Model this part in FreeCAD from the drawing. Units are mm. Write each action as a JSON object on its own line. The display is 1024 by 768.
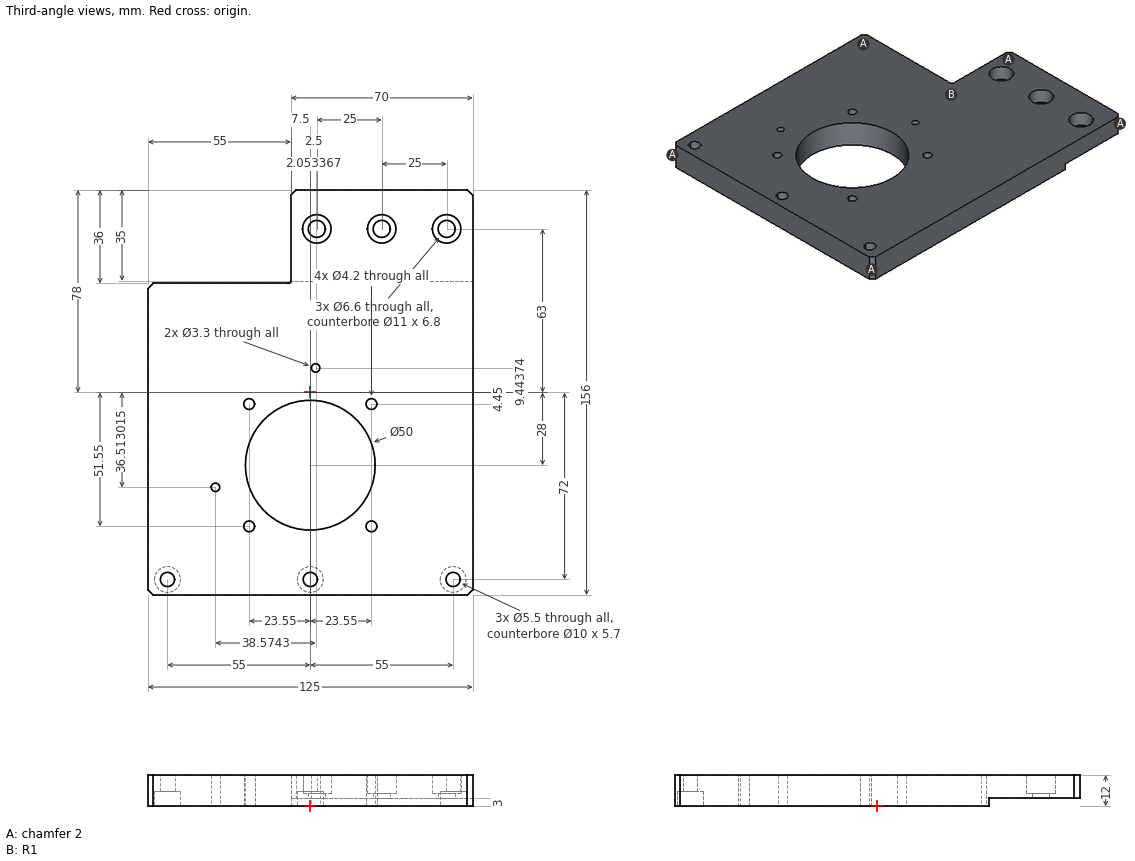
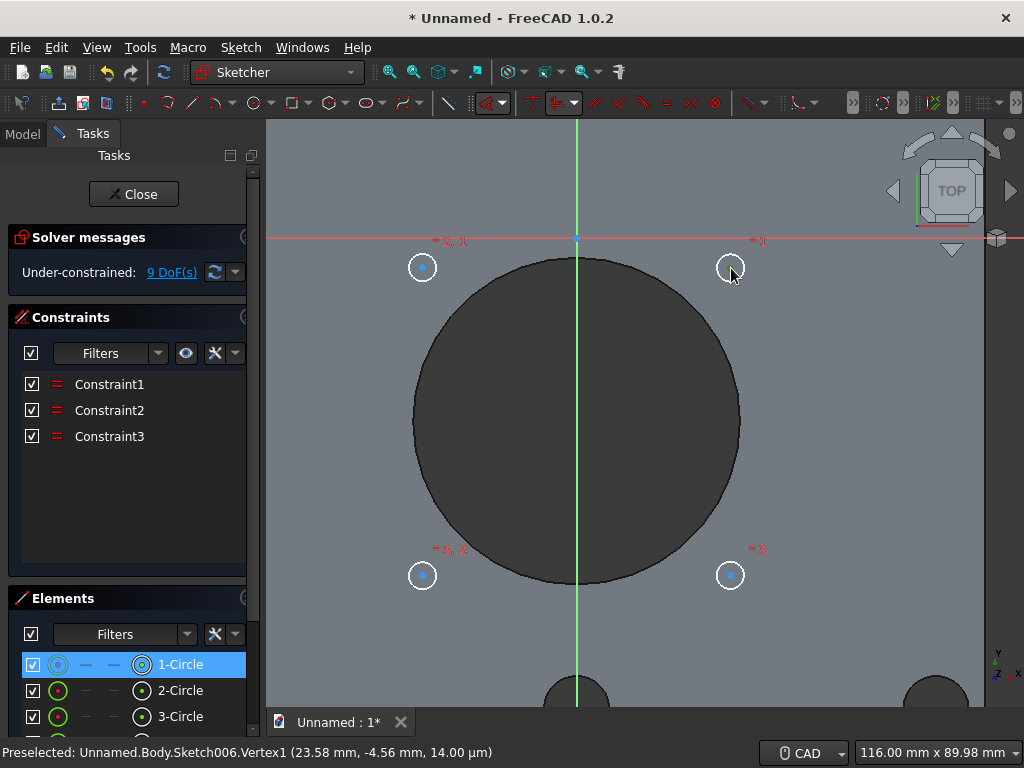
{"action": "left_click", "coordinate": [423, 268]}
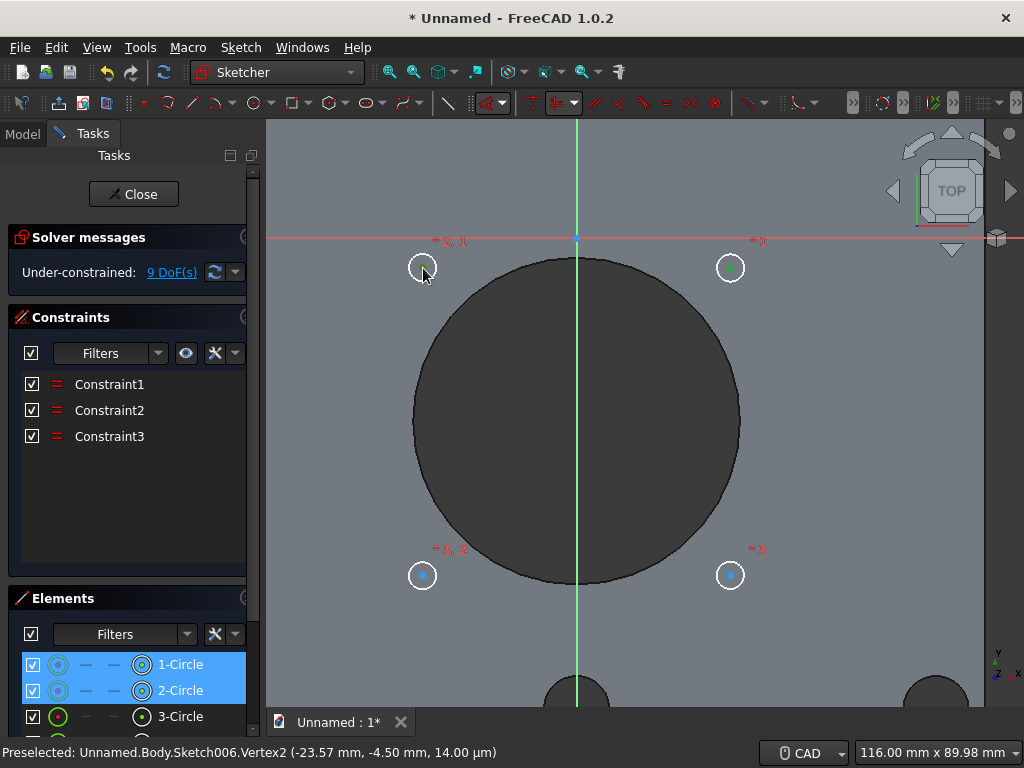
{"action": "left_click", "coordinate": [576, 104]}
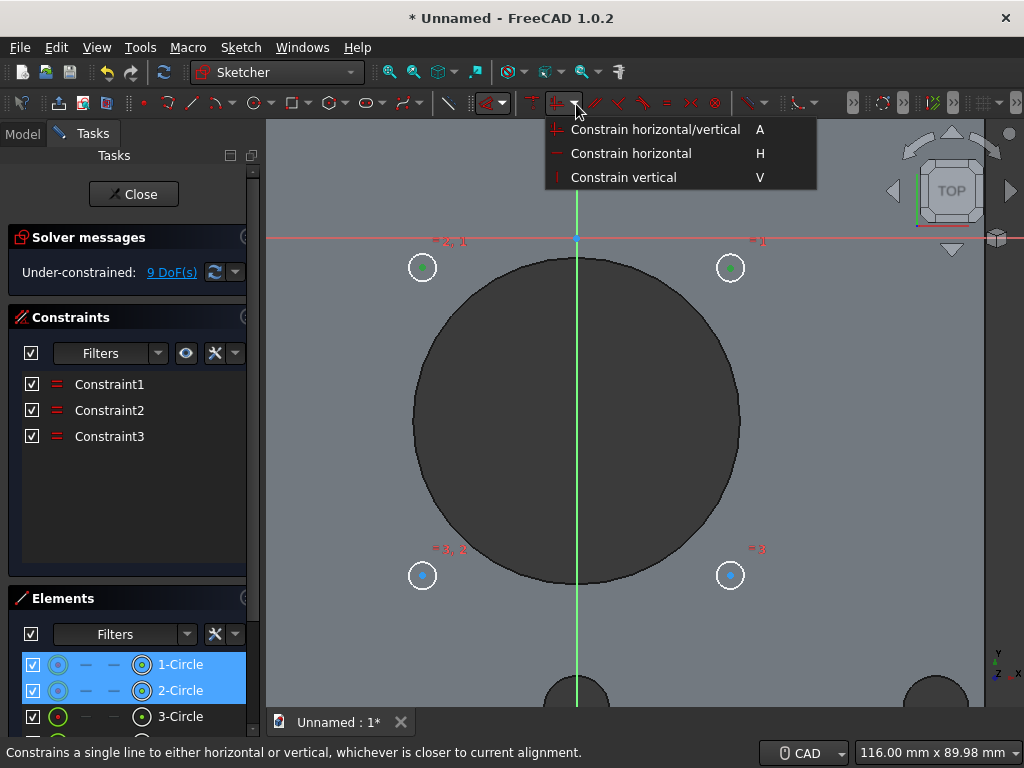
{"action": "left_click", "coordinate": [681, 153]}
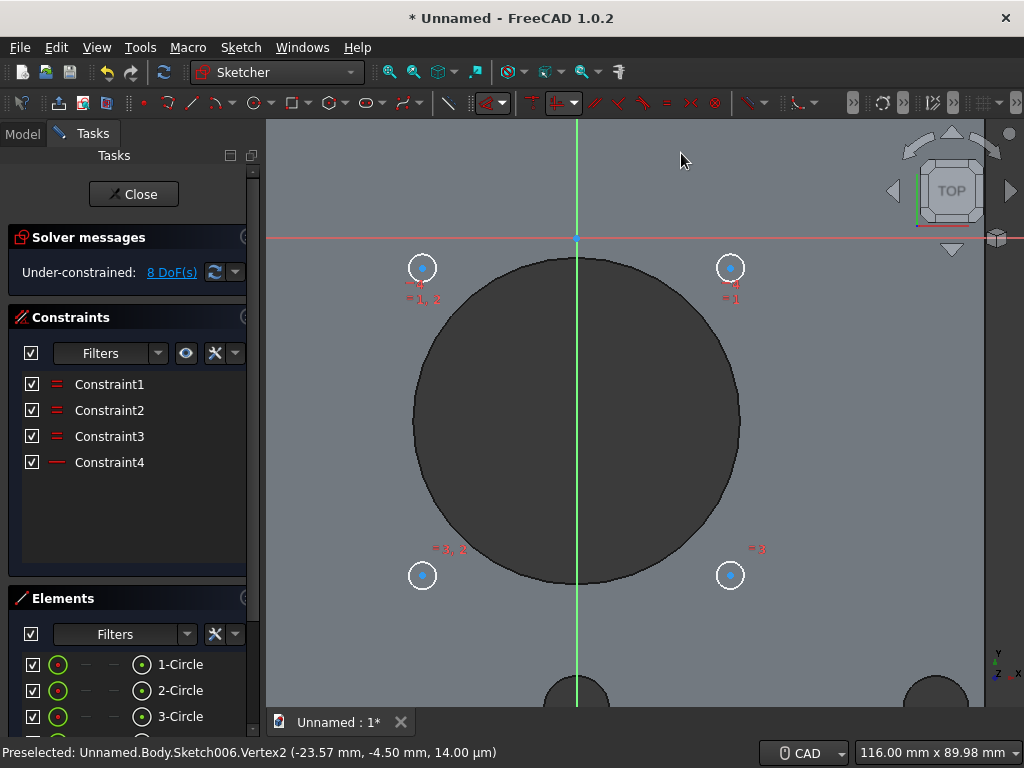
{"action": "left_click", "coordinate": [423, 268]}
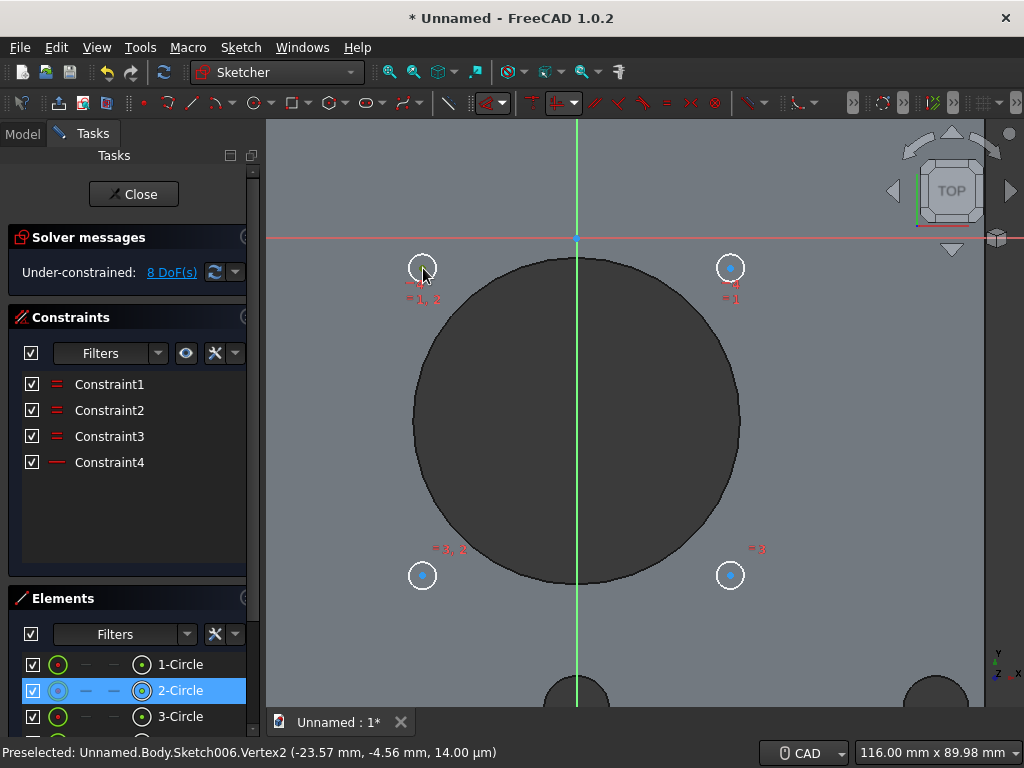
{"action": "left_click", "coordinate": [423, 576]}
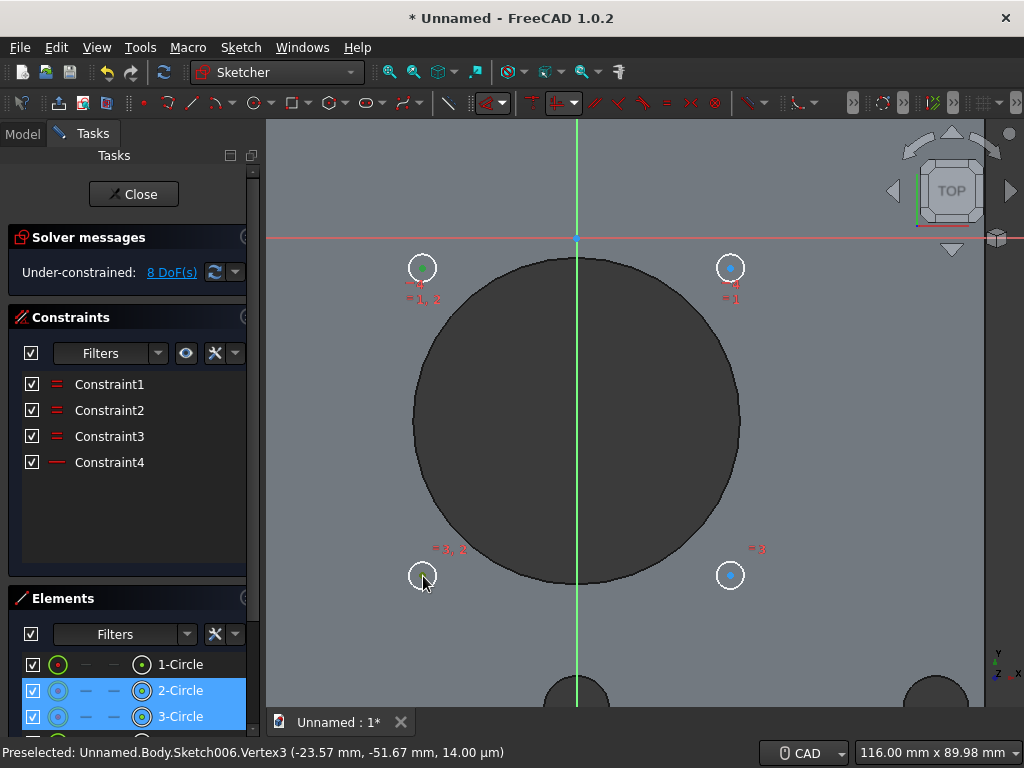
{"action": "left_click", "coordinate": [576, 104]}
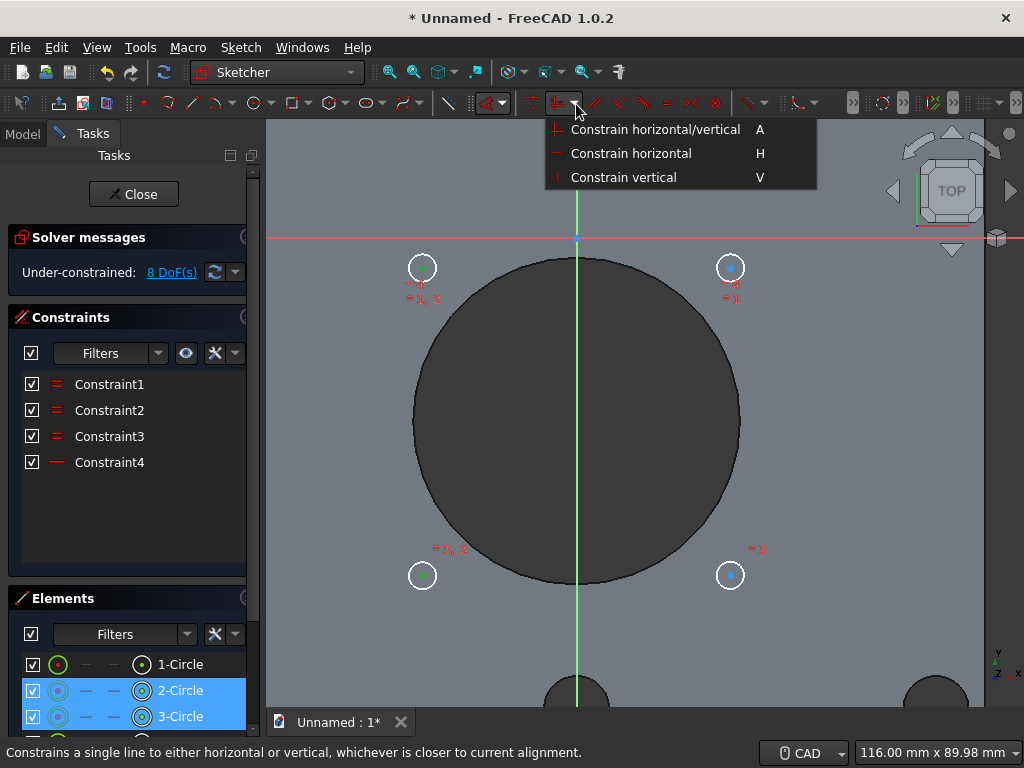
{"action": "left_click", "coordinate": [681, 177]}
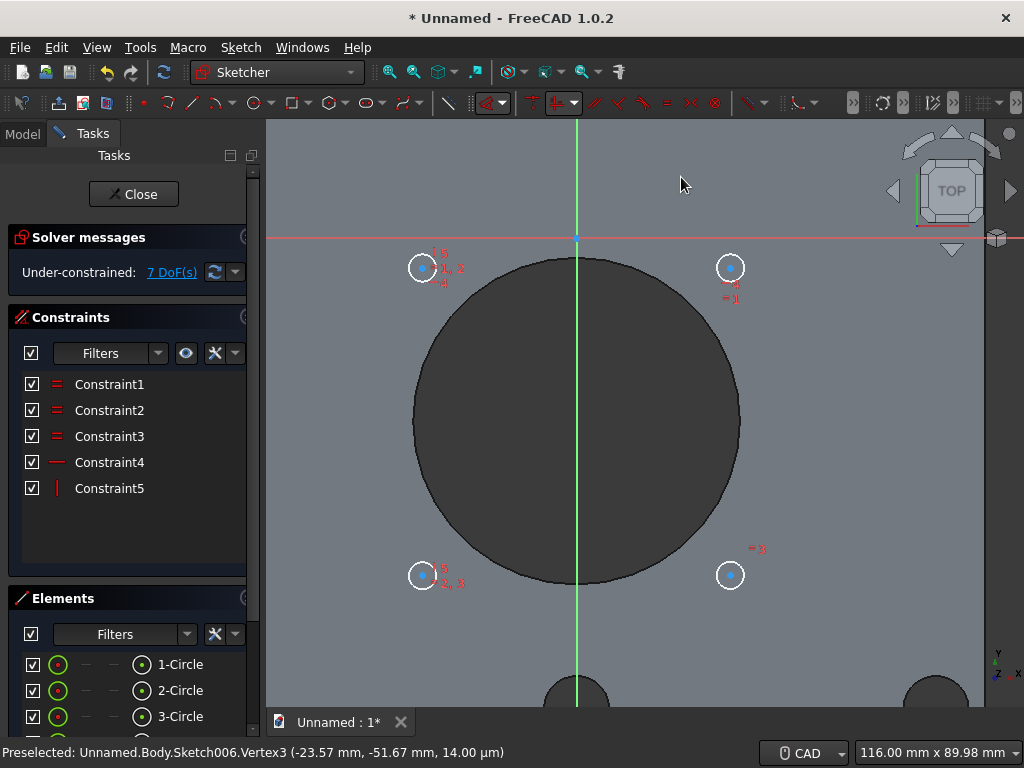
{"action": "left_click", "coordinate": [731, 268]}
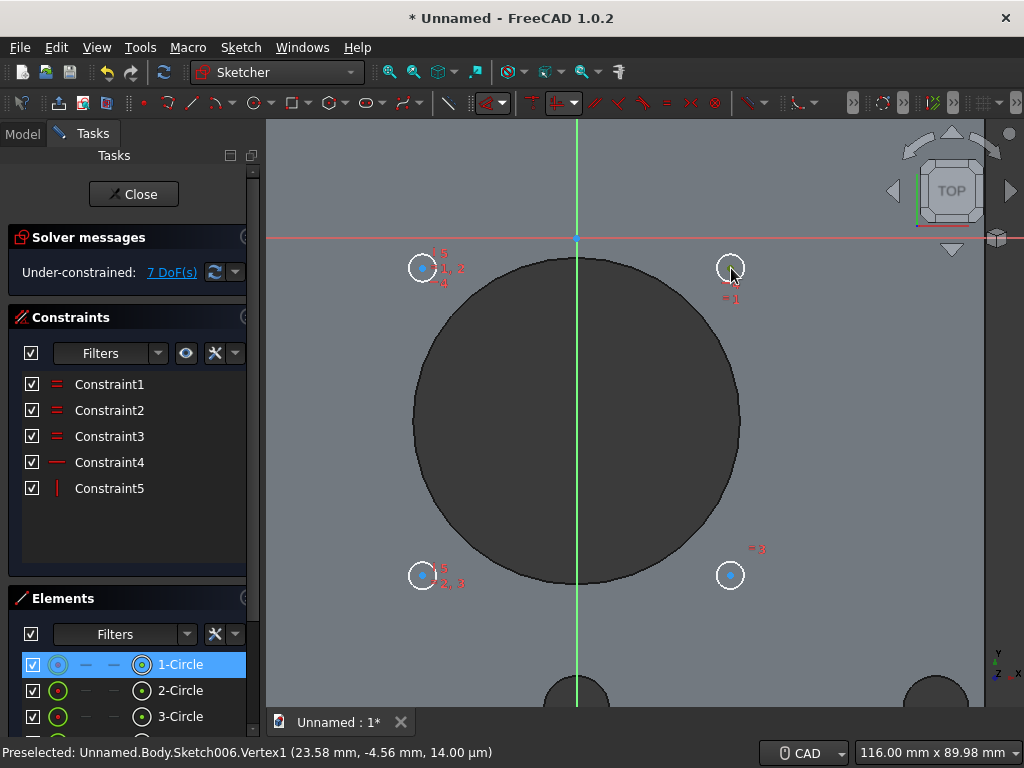
{"action": "left_click", "coordinate": [730, 575]}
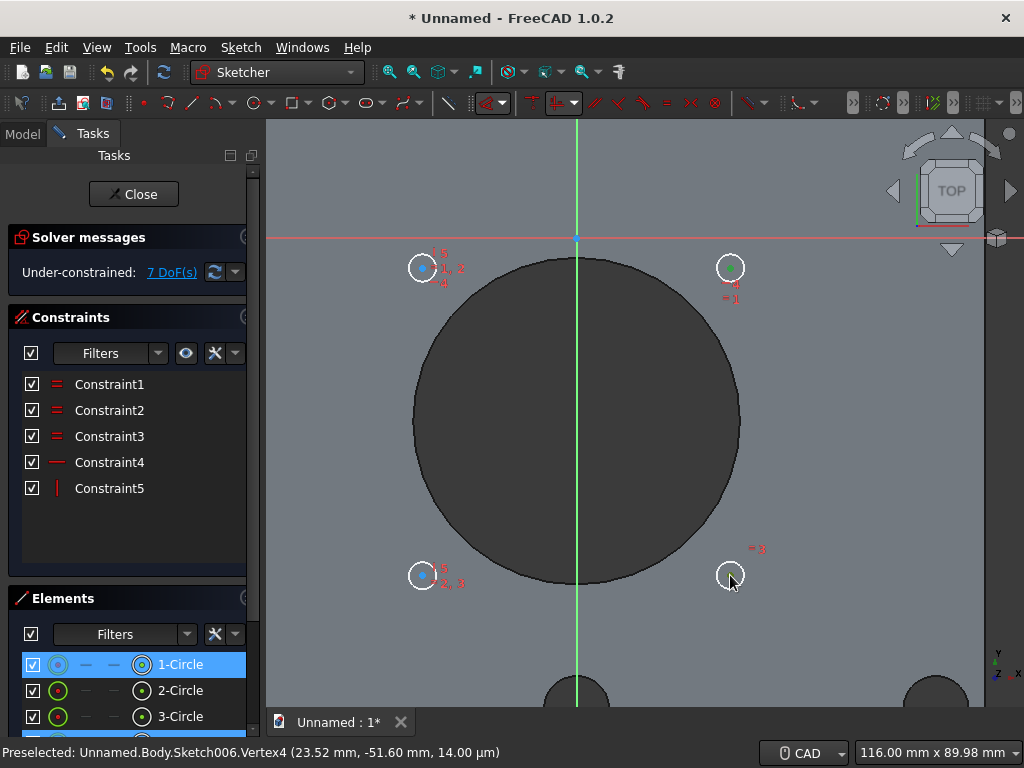
{"action": "key", "text": "v"}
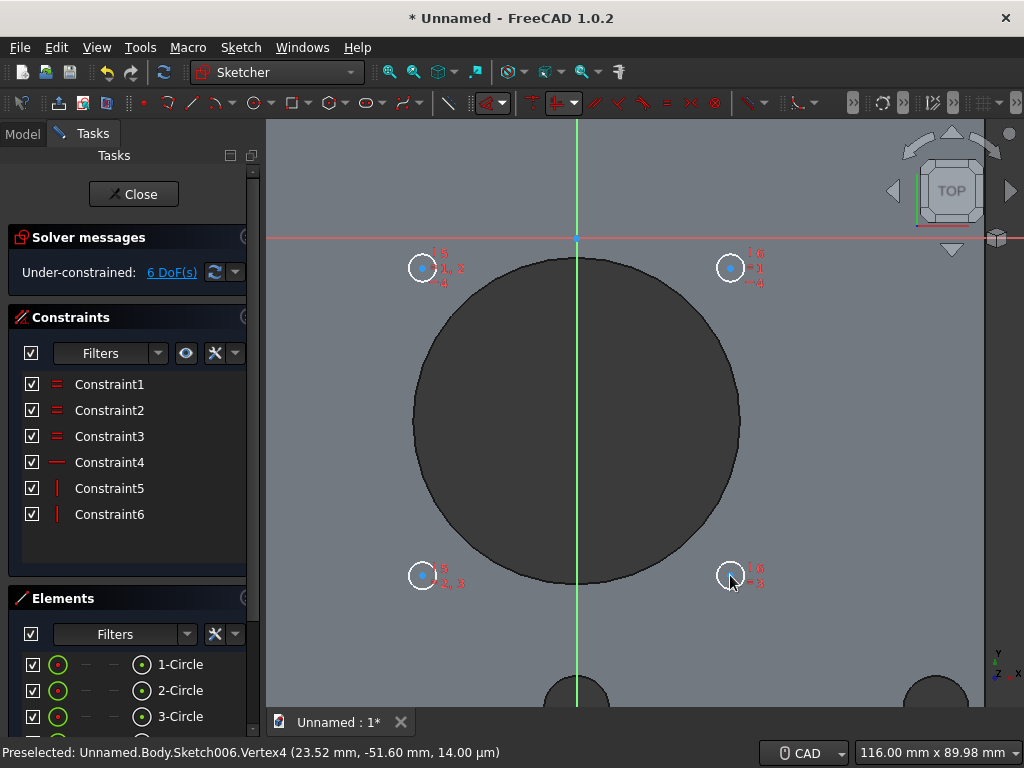
{"action": "left_click", "coordinate": [423, 576]}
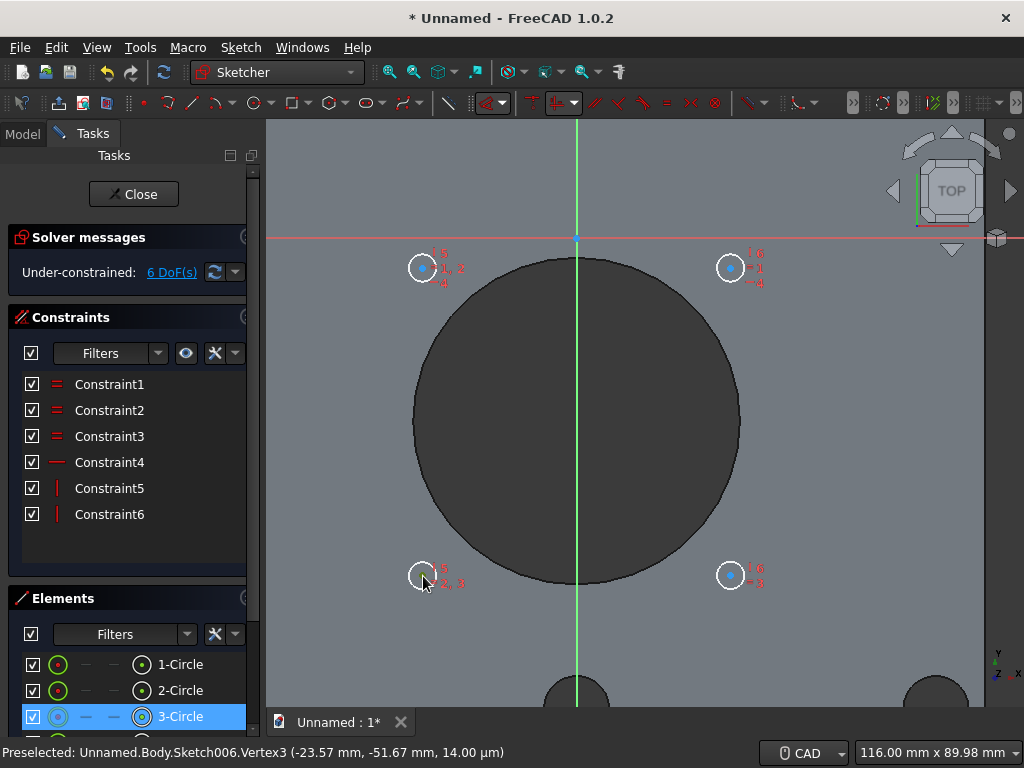
{"action": "left_click", "coordinate": [731, 575]}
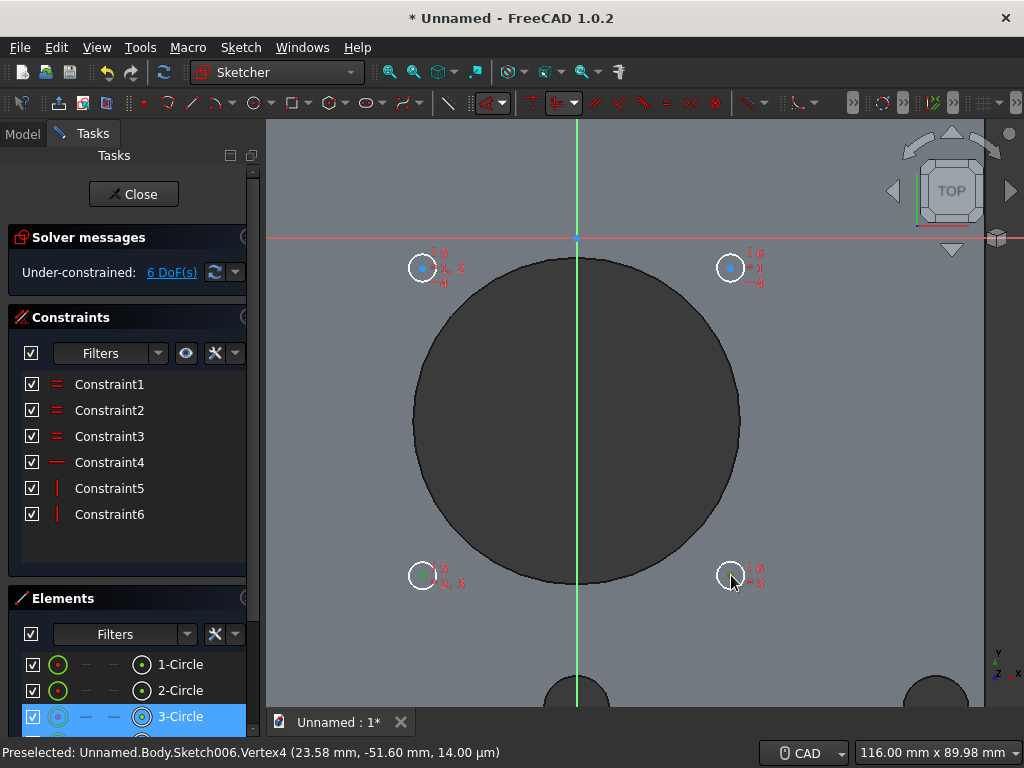
{"action": "left_click", "coordinate": [576, 104]}